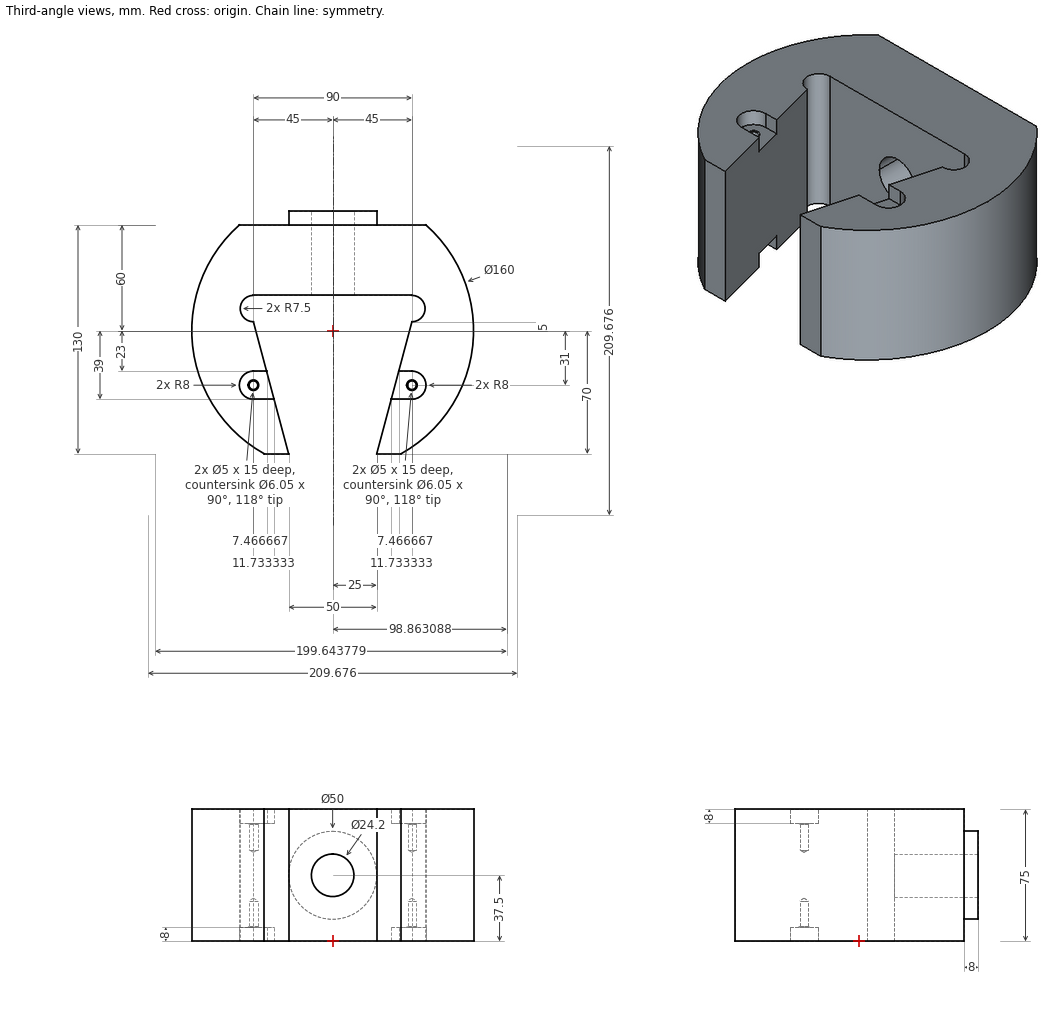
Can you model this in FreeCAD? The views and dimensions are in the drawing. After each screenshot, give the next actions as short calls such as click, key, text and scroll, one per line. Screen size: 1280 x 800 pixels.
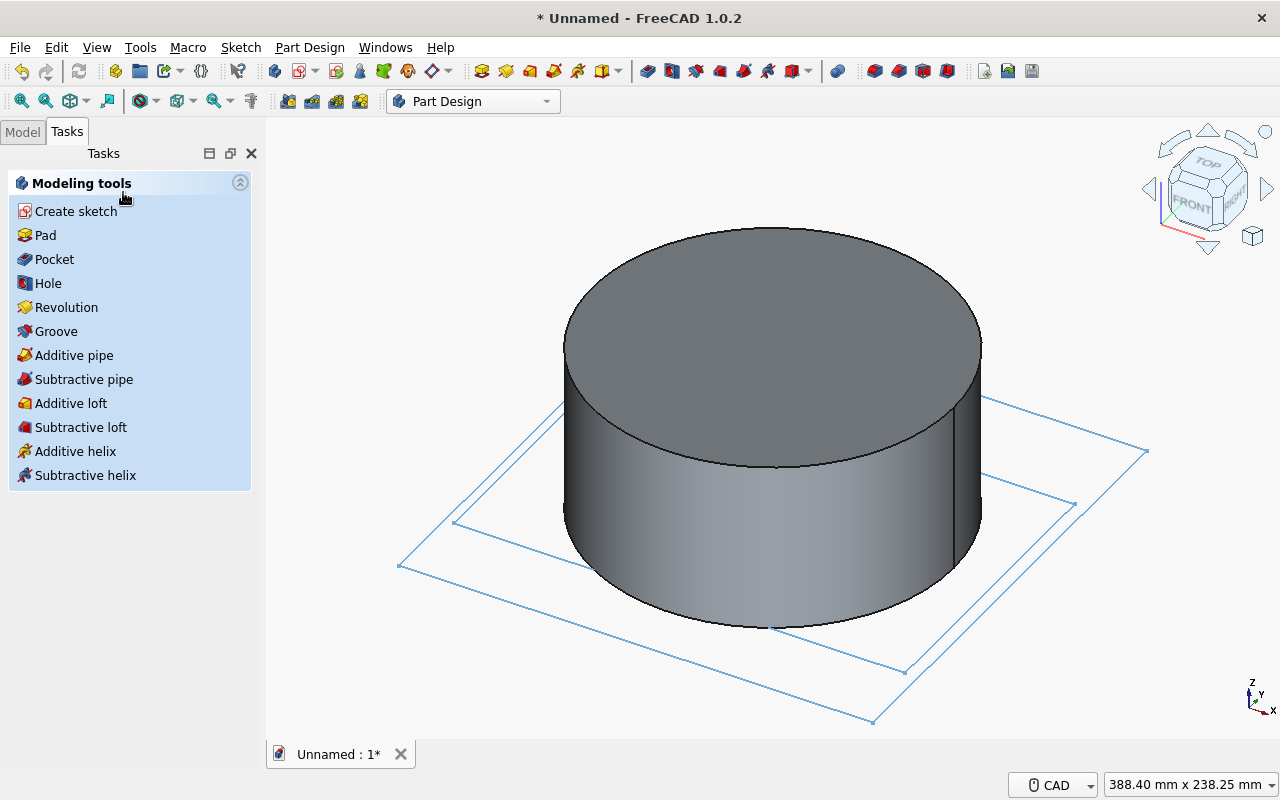
click(648, 72)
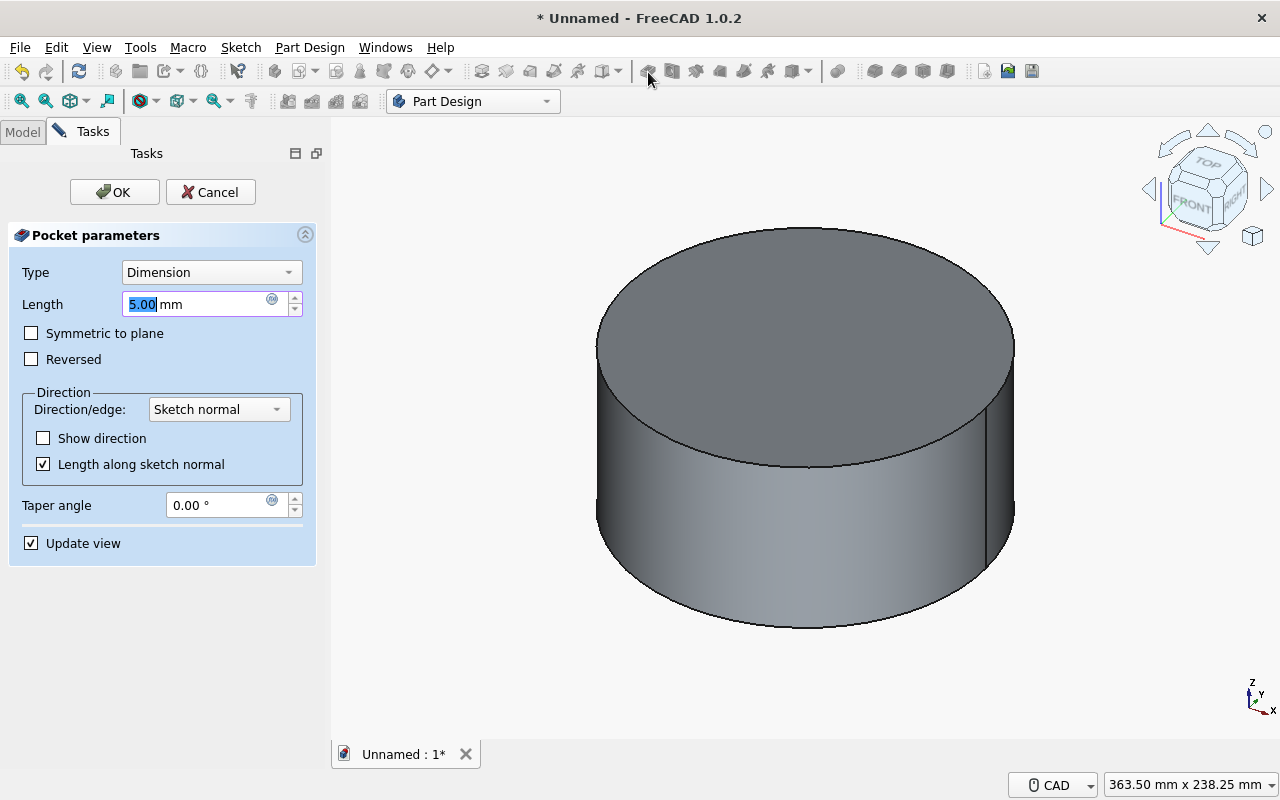
click(212, 272)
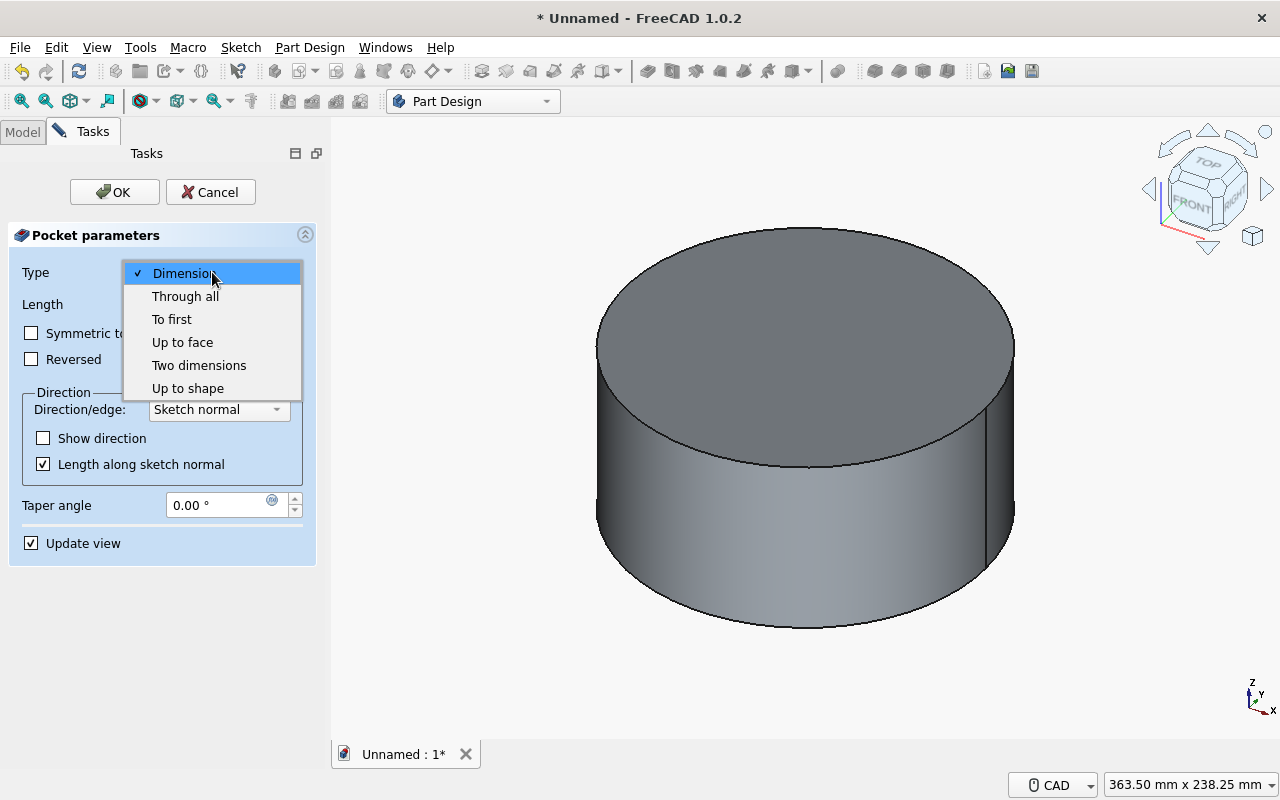
click(212, 296)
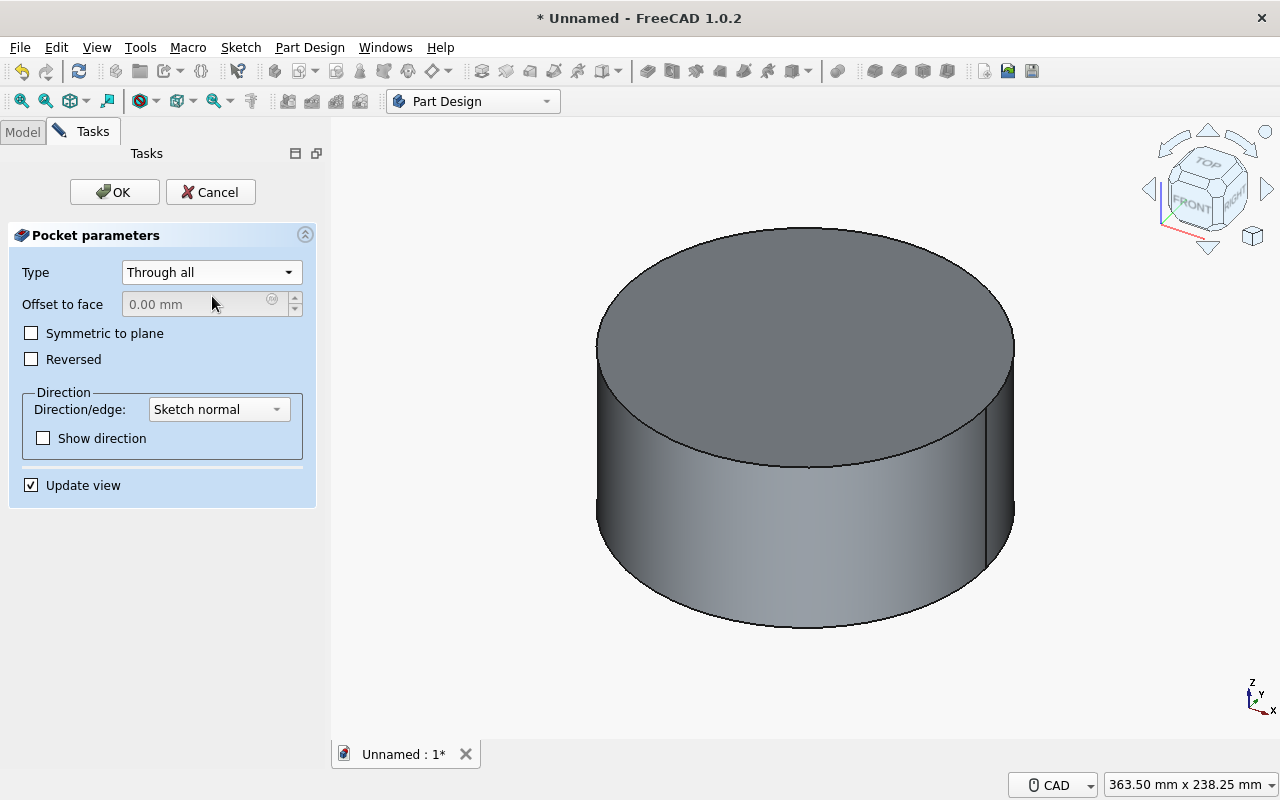
click(30, 359)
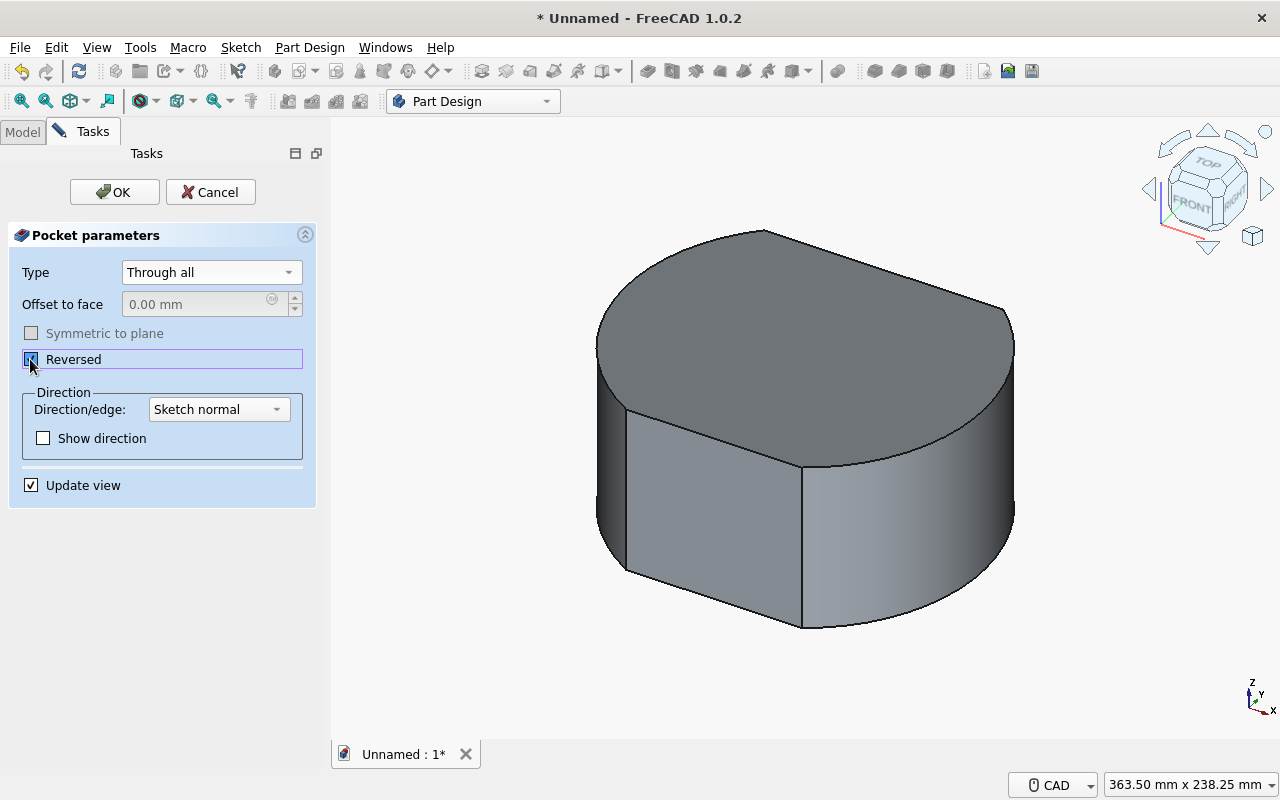
click(115, 192)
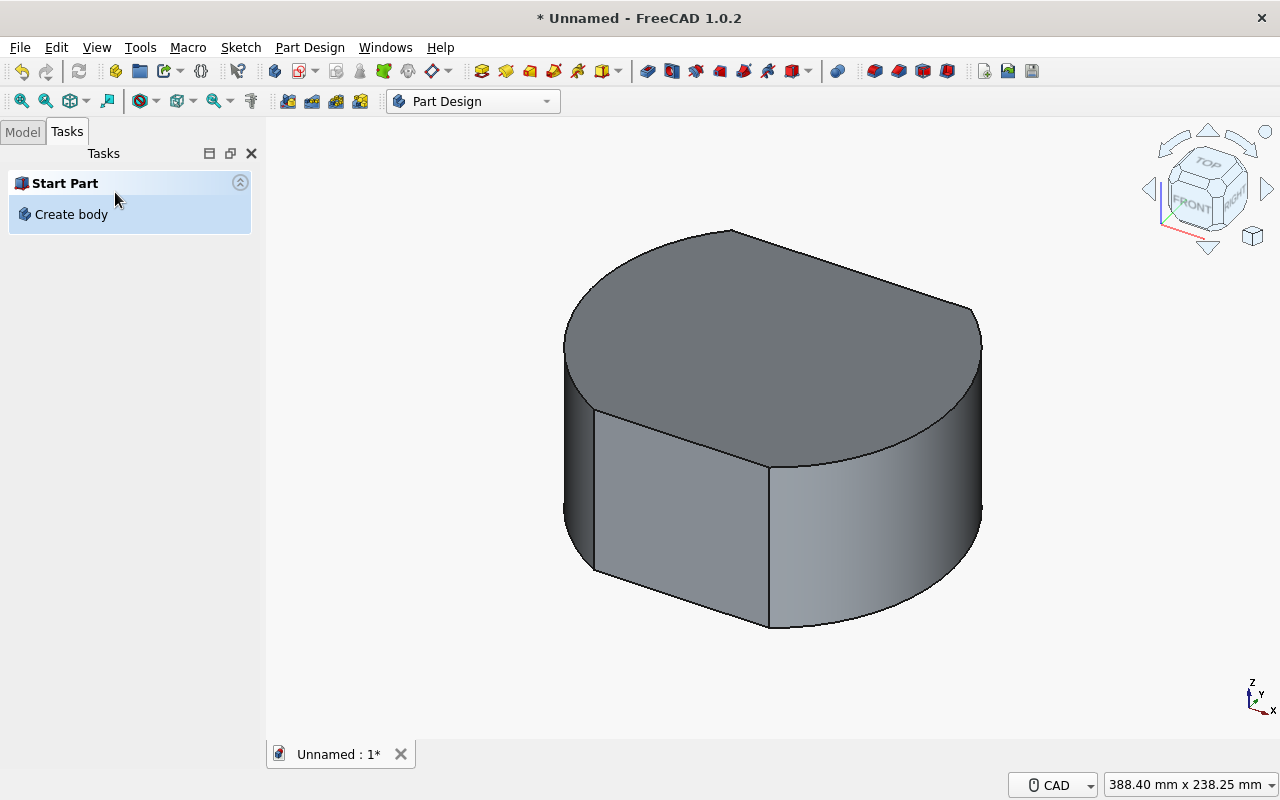
click(300, 72)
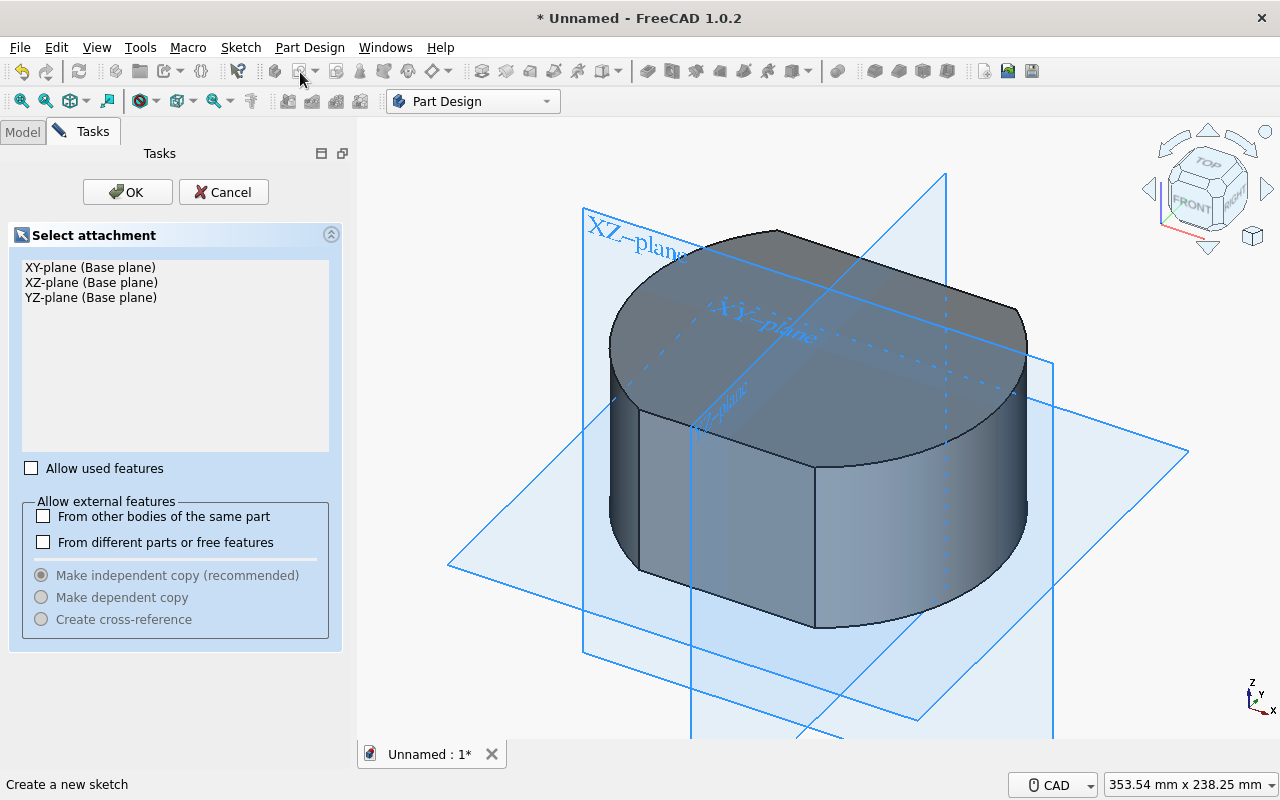
click(82, 268)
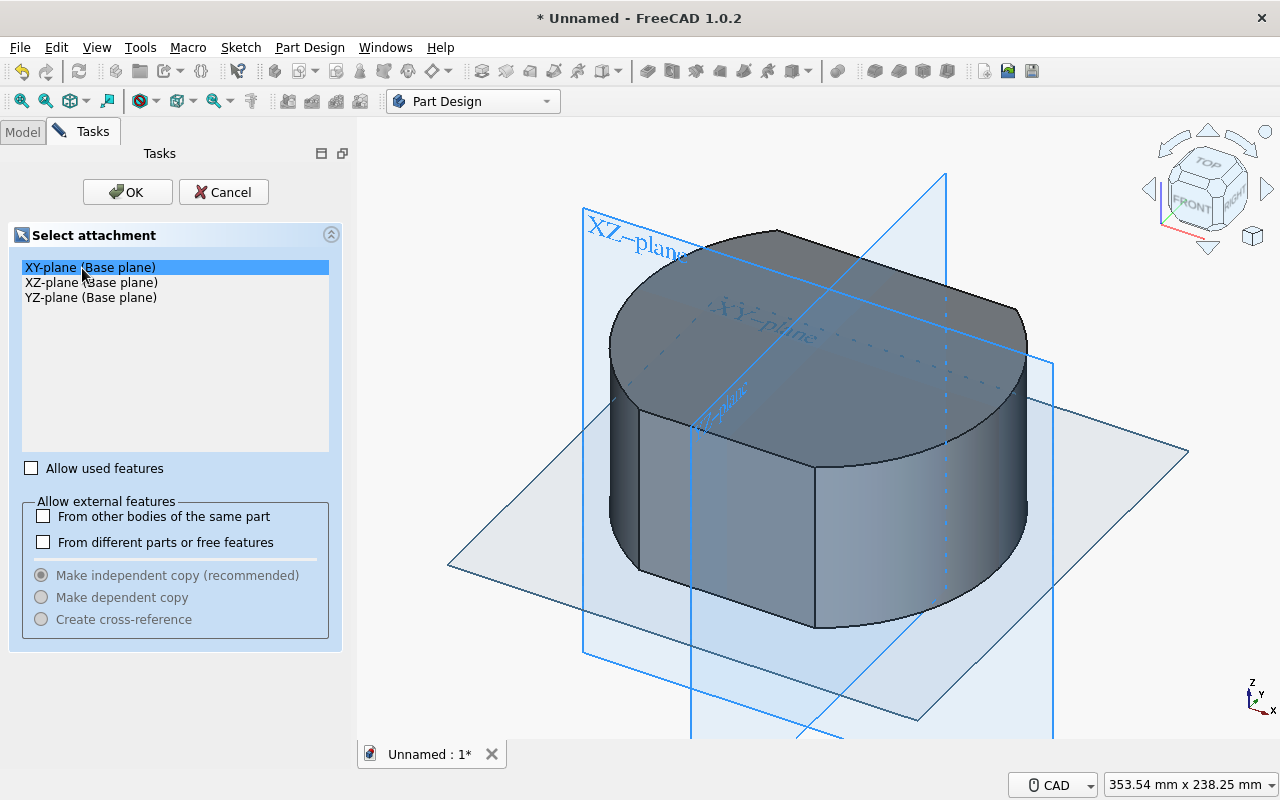
click(128, 192)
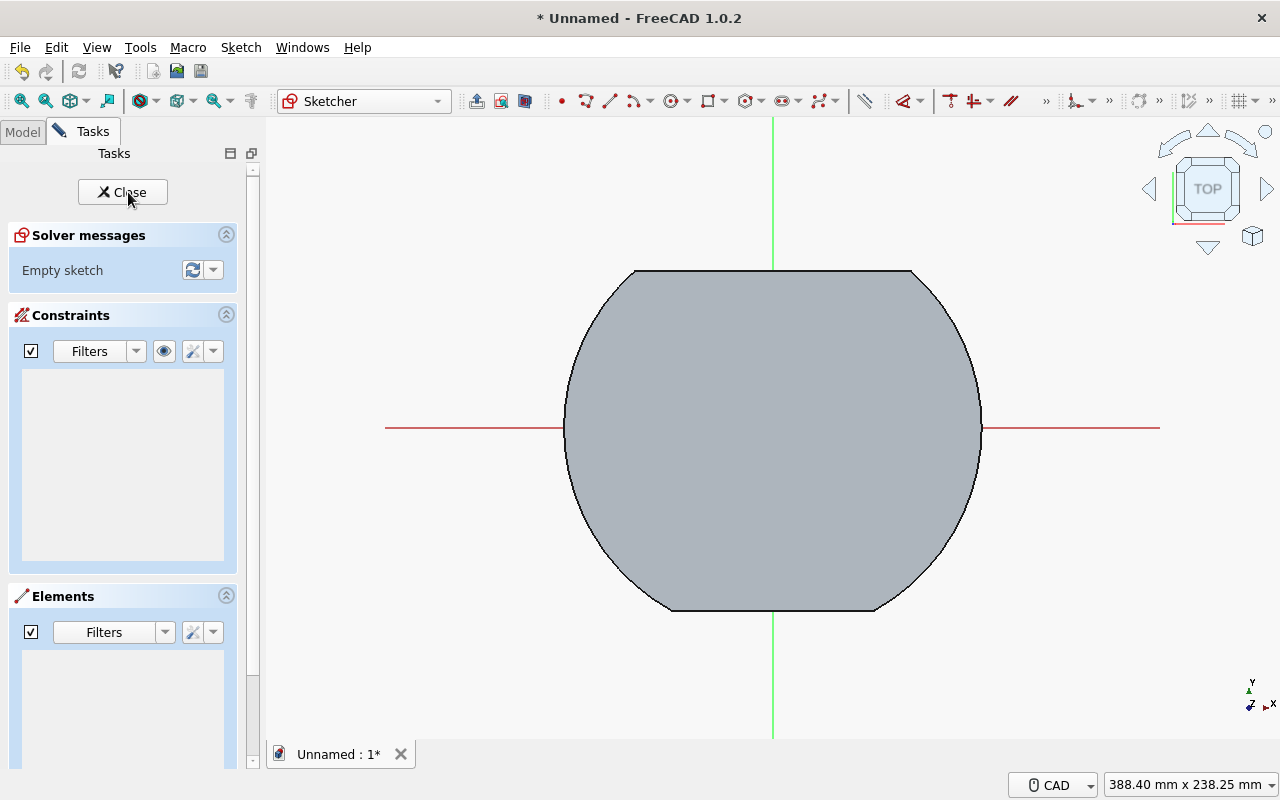
key(q)
key(s)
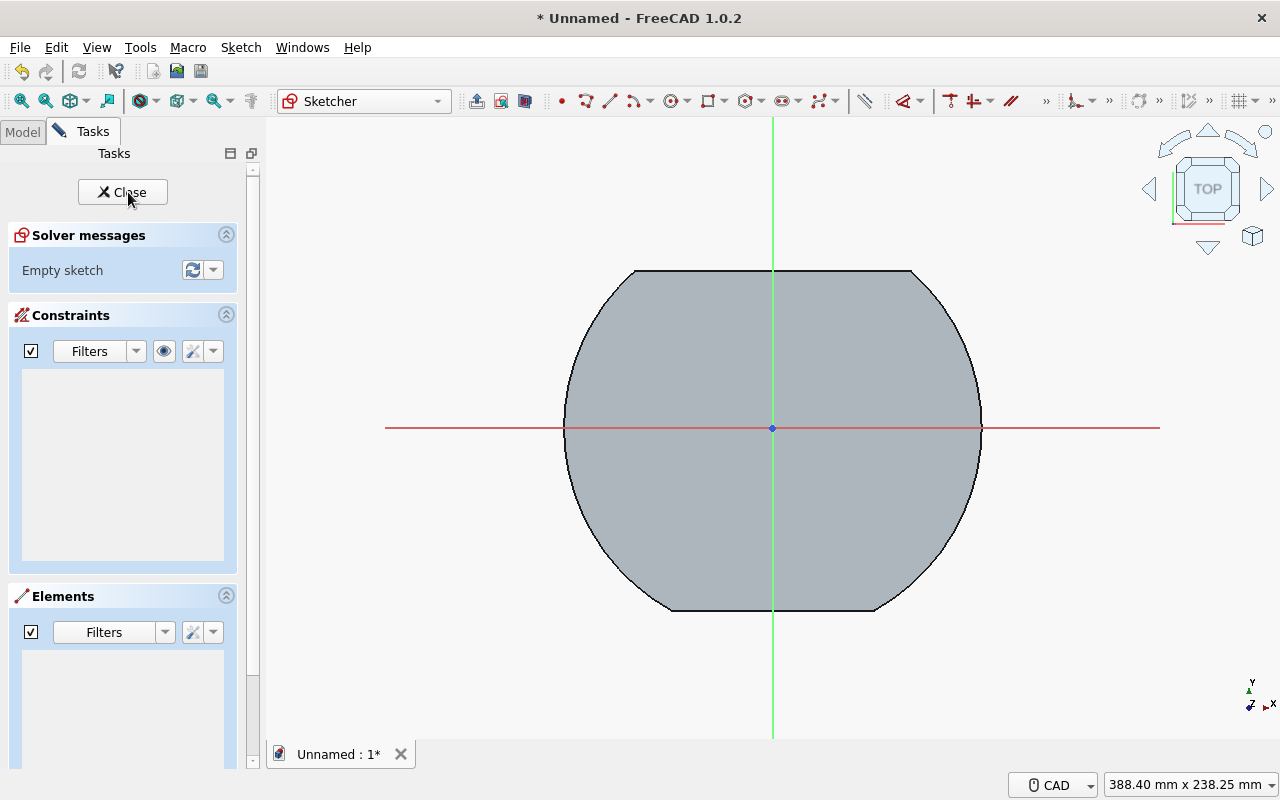
scroll(856, 573, up, 3)